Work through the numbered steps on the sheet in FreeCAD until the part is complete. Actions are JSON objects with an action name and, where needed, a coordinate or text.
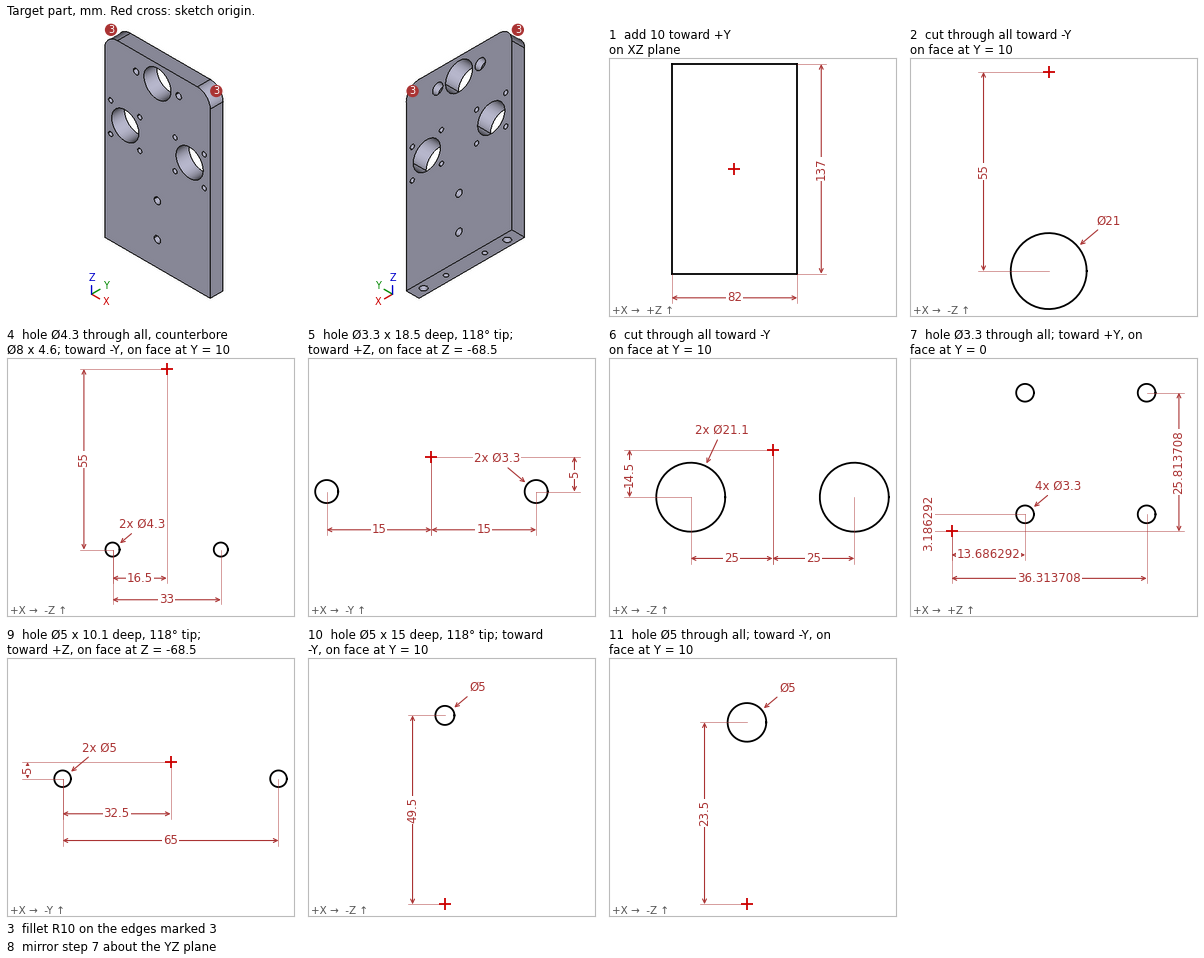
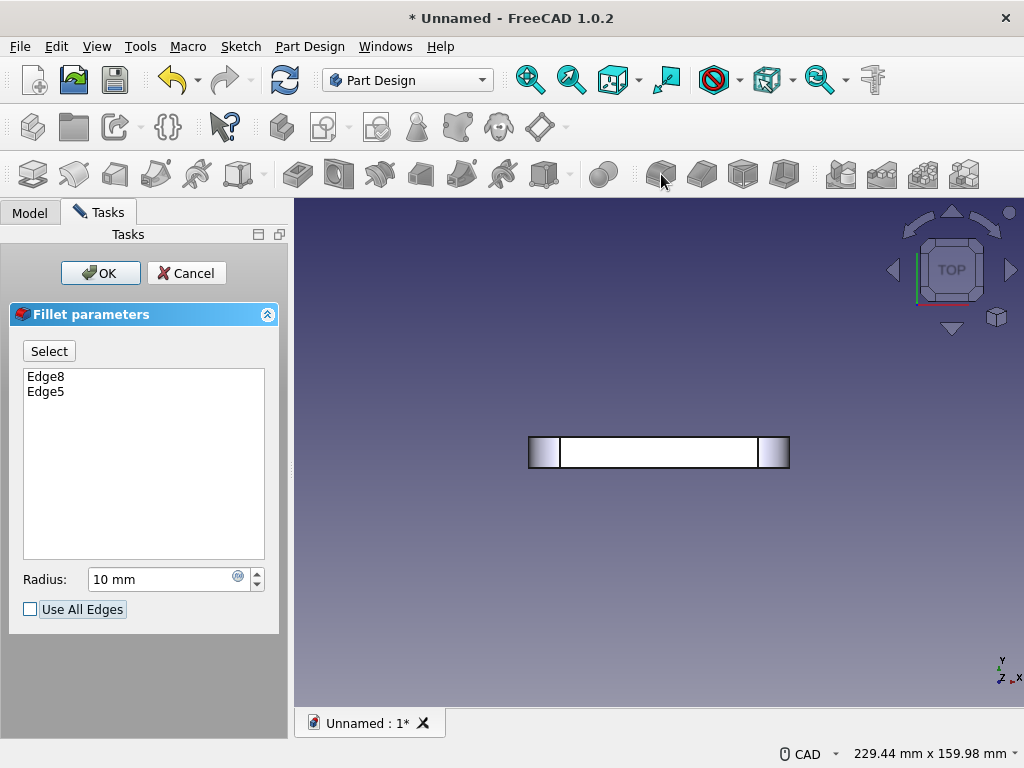
{"action": "left_click", "coordinate": [101, 273]}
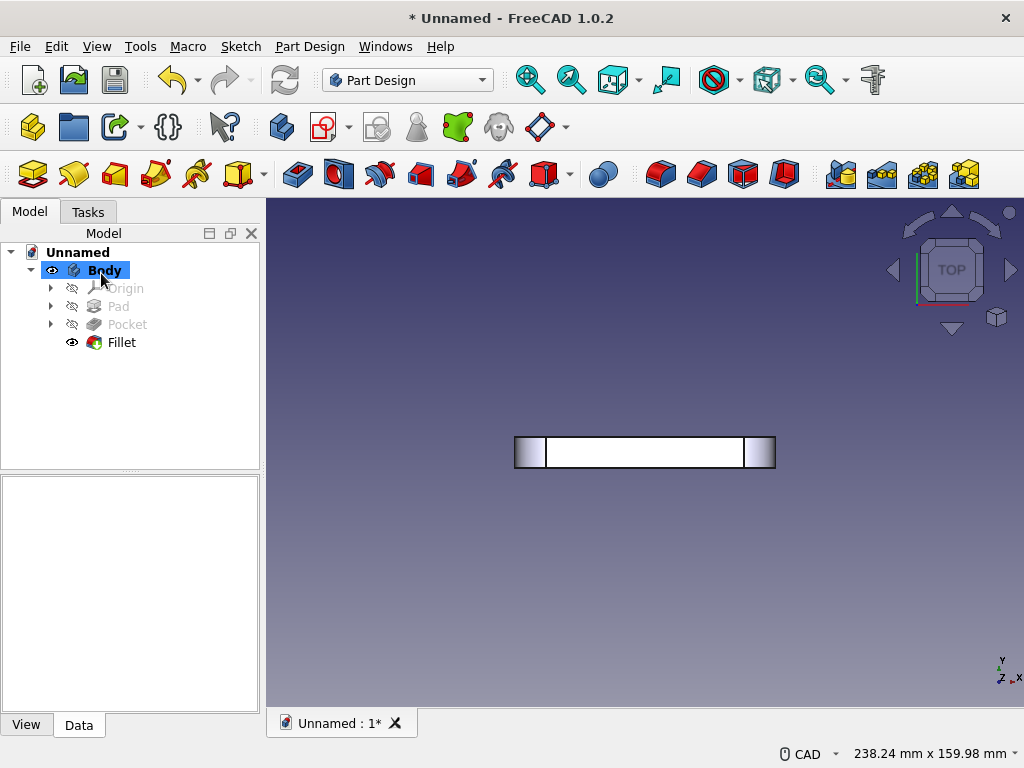
{"action": "left_click", "coordinate": [531, 80]}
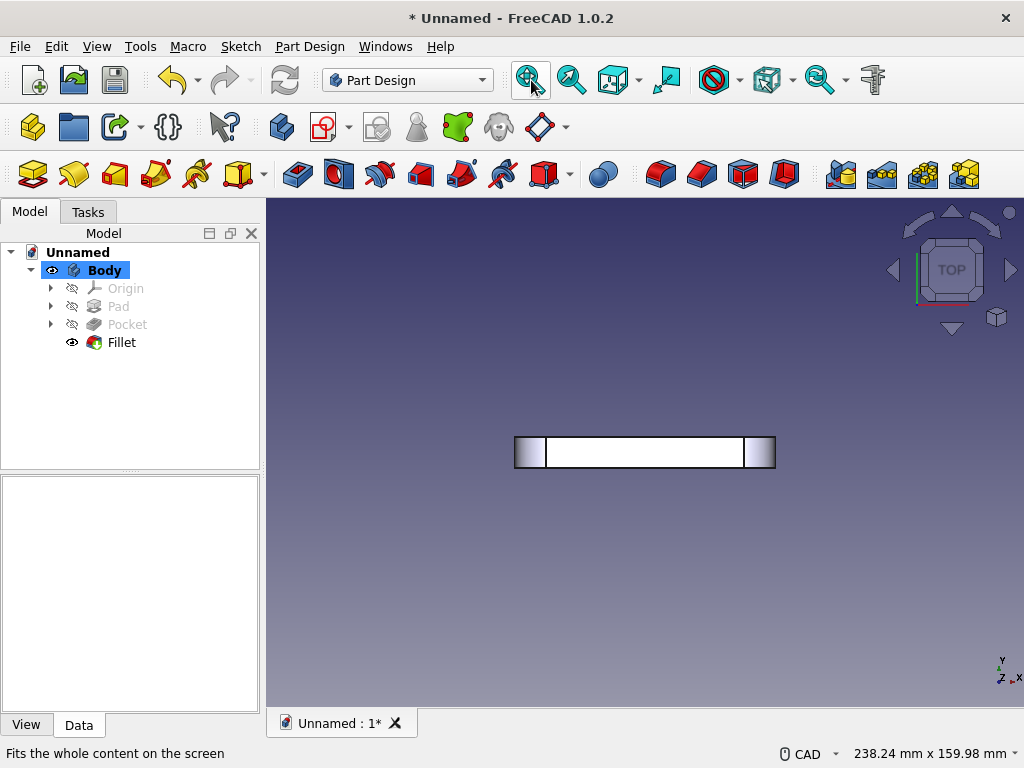
{"action": "key", "text": "4"}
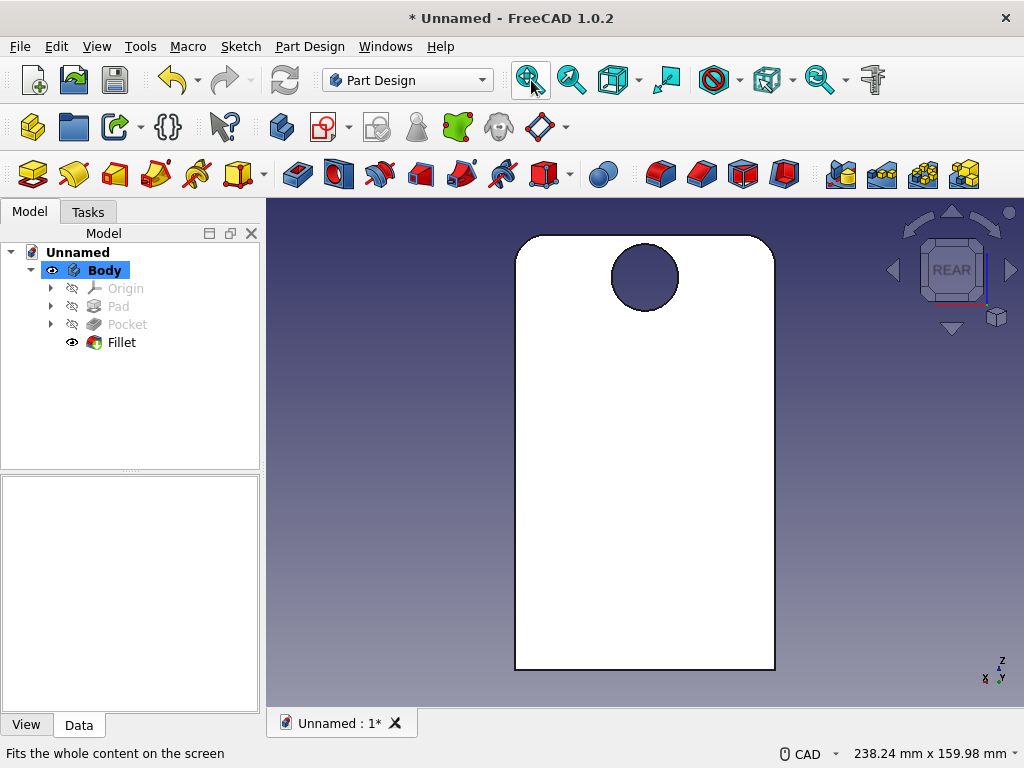
{"action": "left_click", "coordinate": [645, 451]}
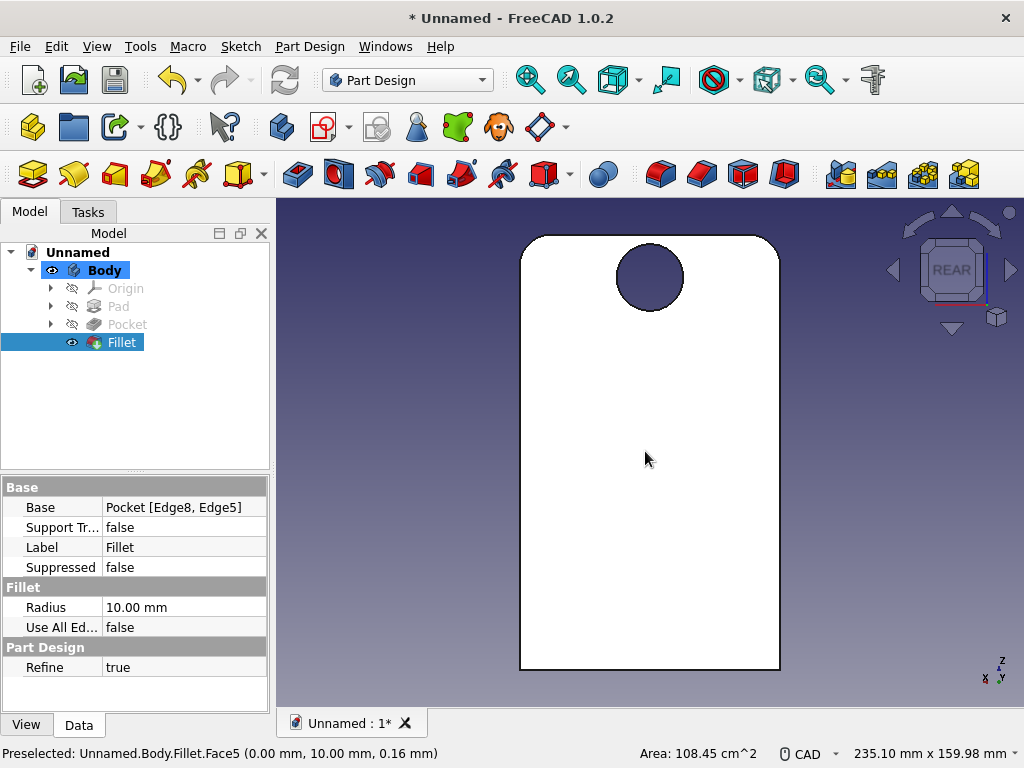
{"action": "left_click", "coordinate": [322, 128]}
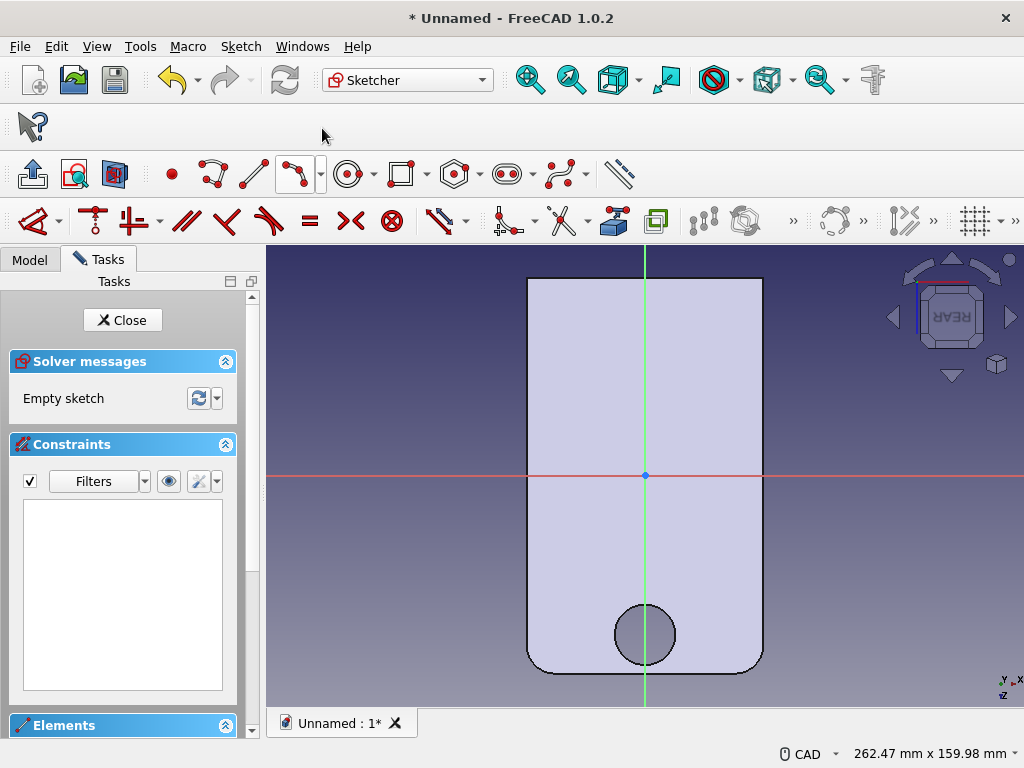
{"action": "scroll", "coordinate": [728, 659], "scroll_direction": "up", "scroll_amount": 3}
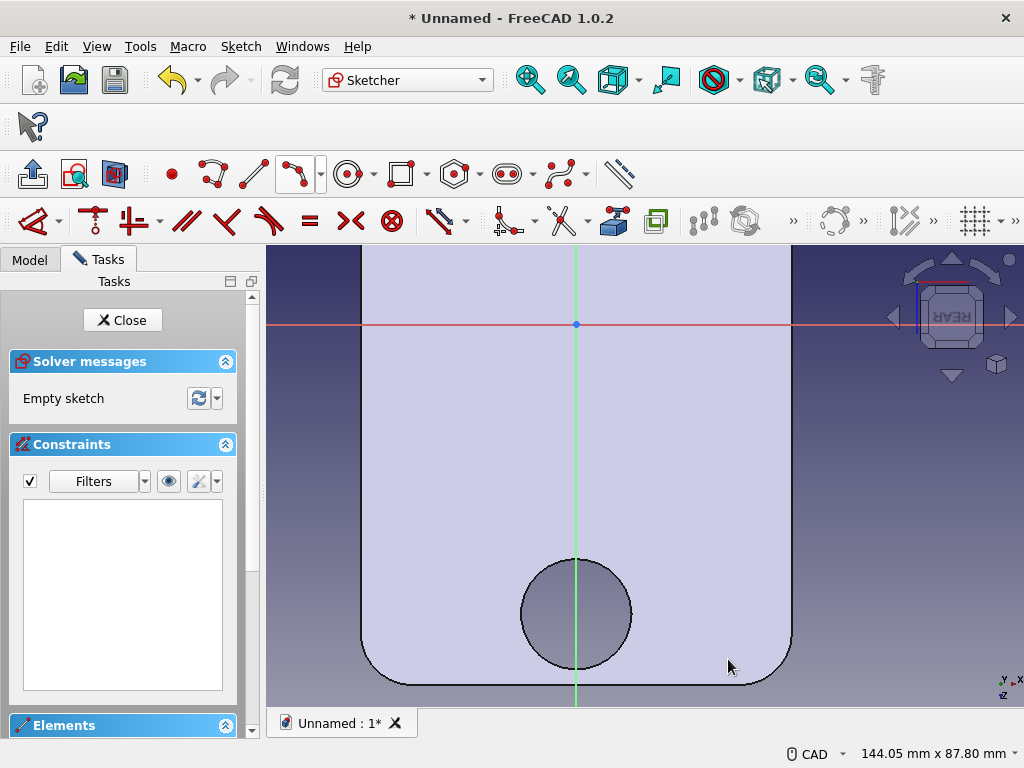
{"action": "key", "text": "g c"}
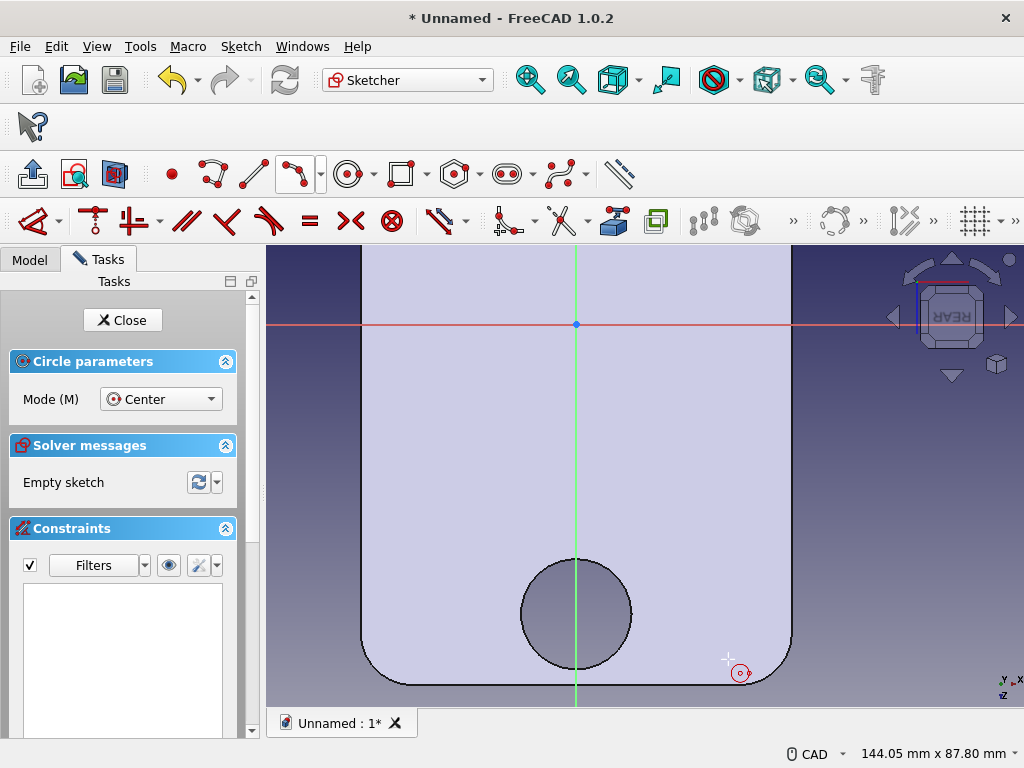
{"action": "scroll", "coordinate": [489, 614], "scroll_direction": "up", "scroll_amount": 4}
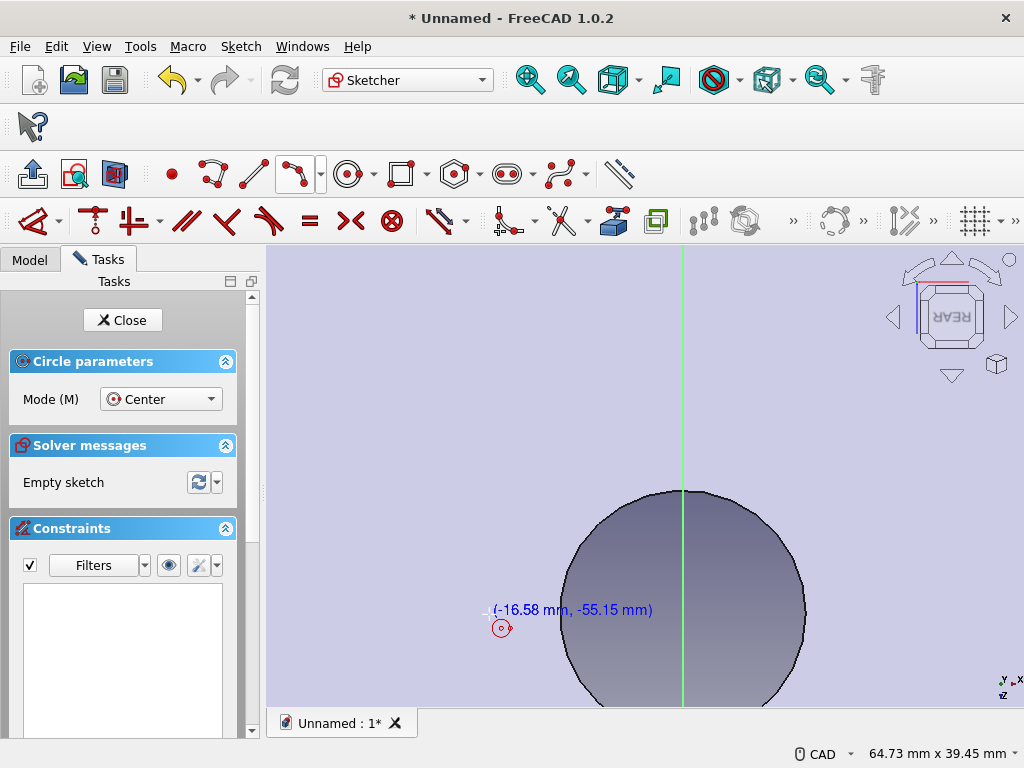
{"action": "left_click", "coordinate": [490, 614]}
{"action": "mouse_move", "coordinate": [507, 596]}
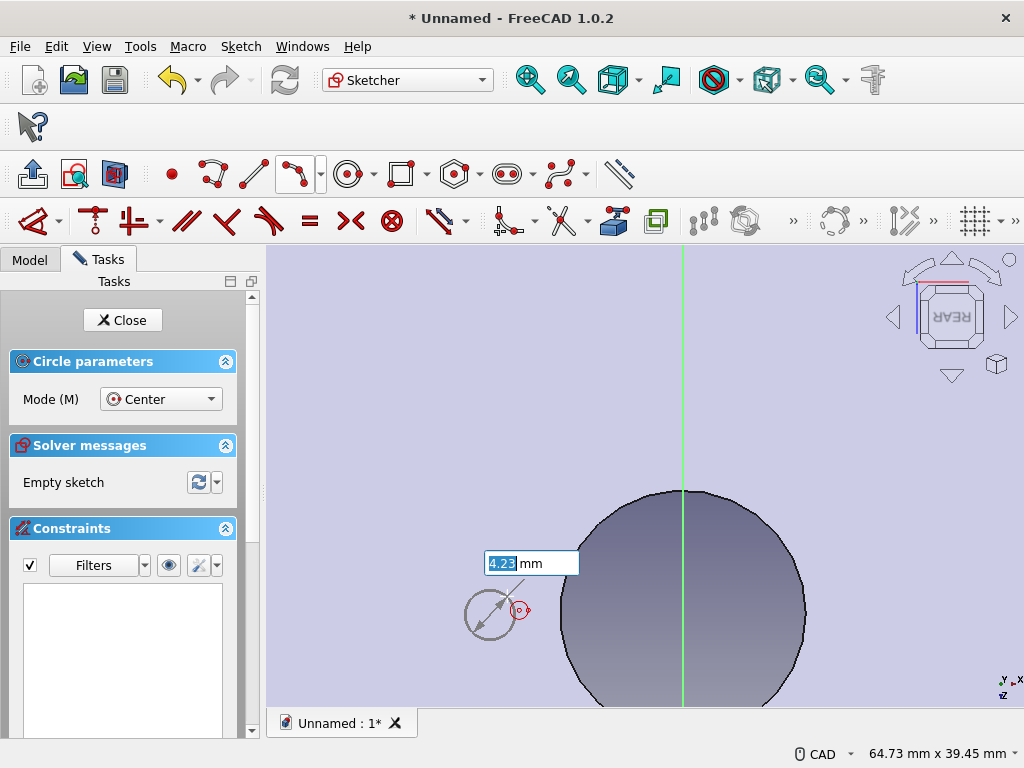
{"action": "type", "text": "4.3"}
{"action": "key", "text": "Return"}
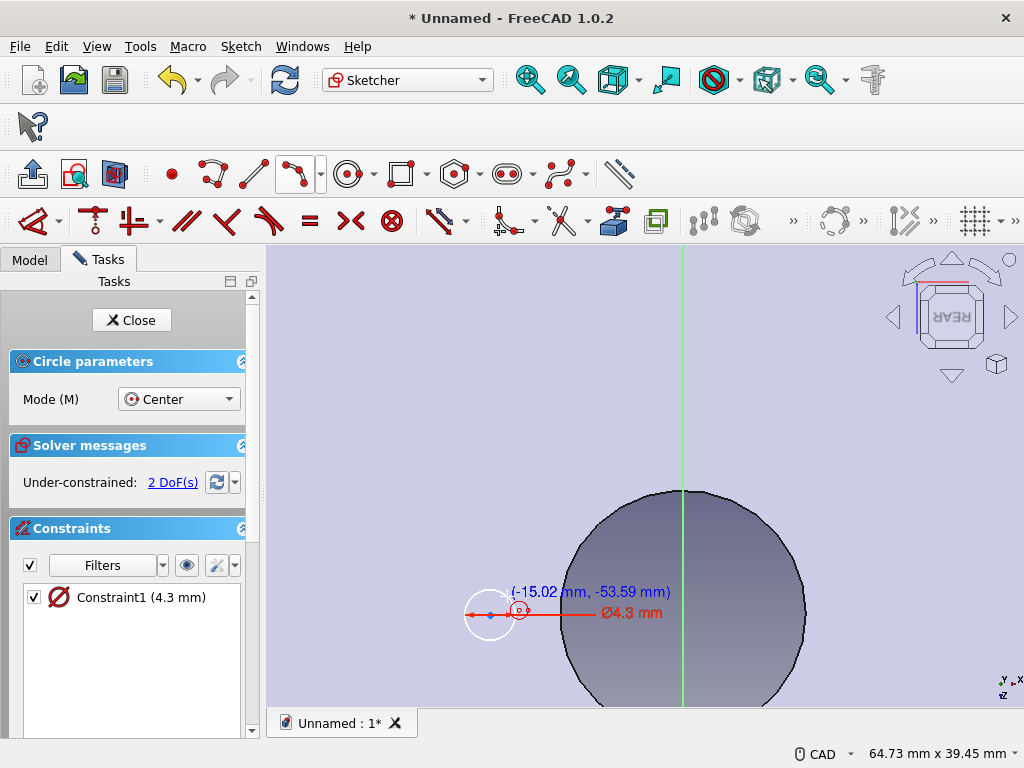
{"action": "scroll", "coordinate": [490, 616], "scroll_direction": "down", "scroll_amount": 4}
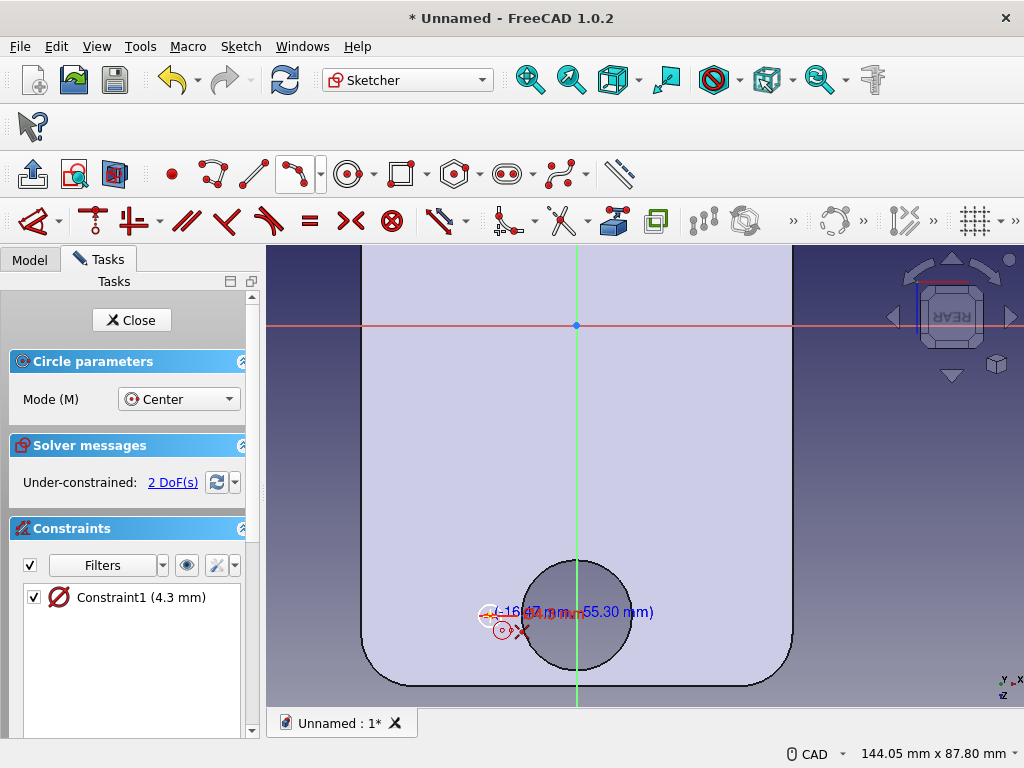
{"action": "scroll", "coordinate": [664, 615], "scroll_direction": "up", "scroll_amount": 4}